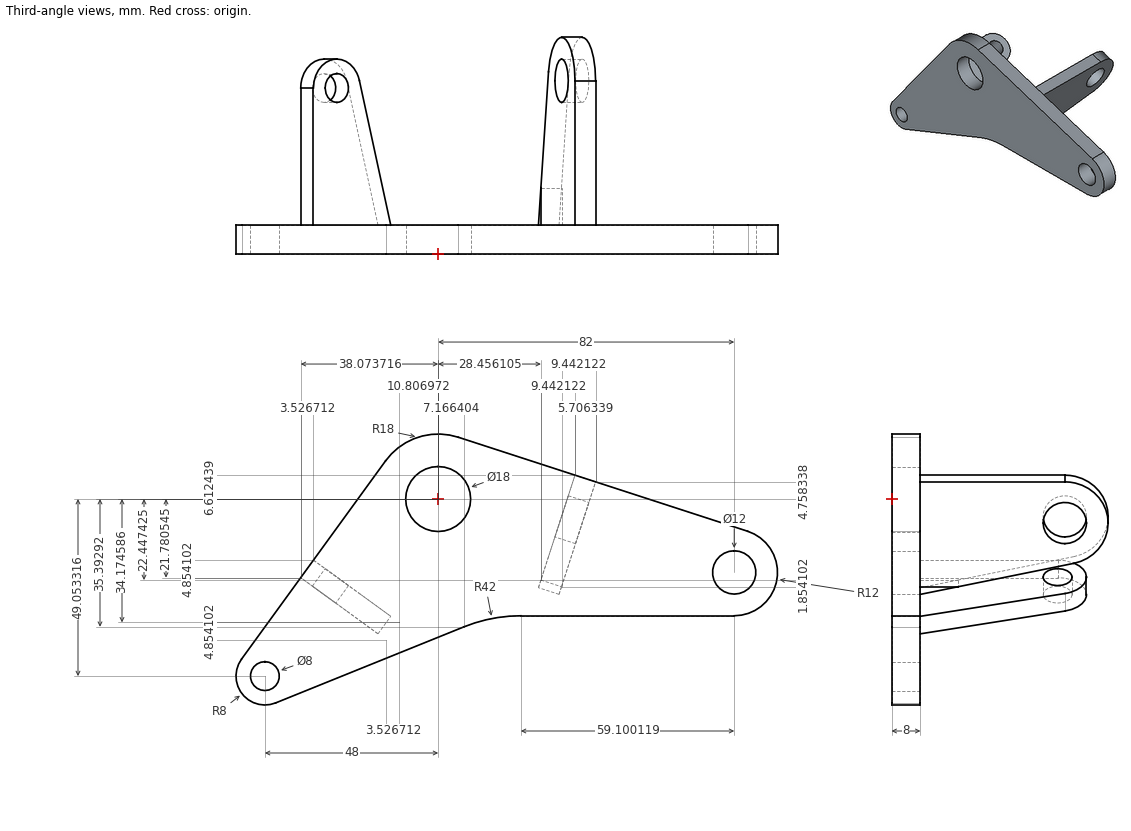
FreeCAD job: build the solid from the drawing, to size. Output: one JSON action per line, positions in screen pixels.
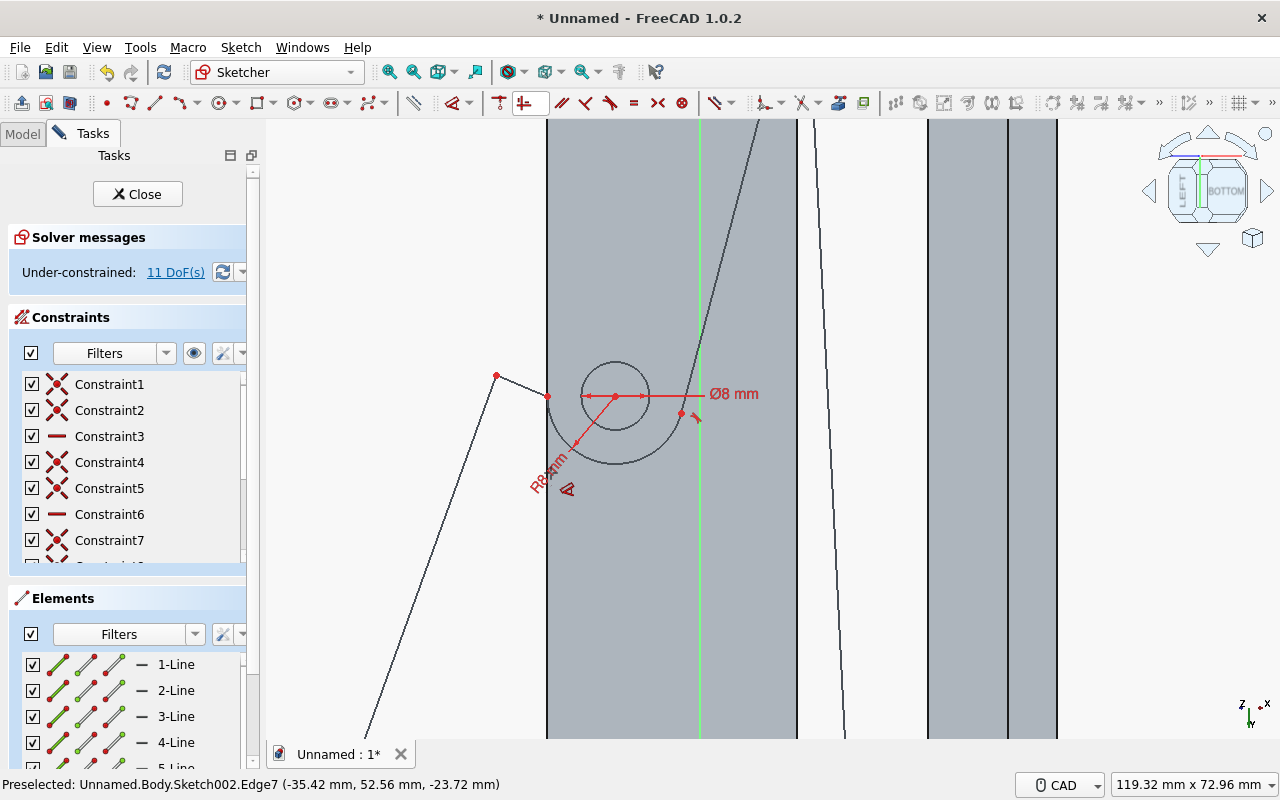
{"action": "scroll", "coordinate": [812, 393], "scroll_direction": "down", "scroll_amount": 4}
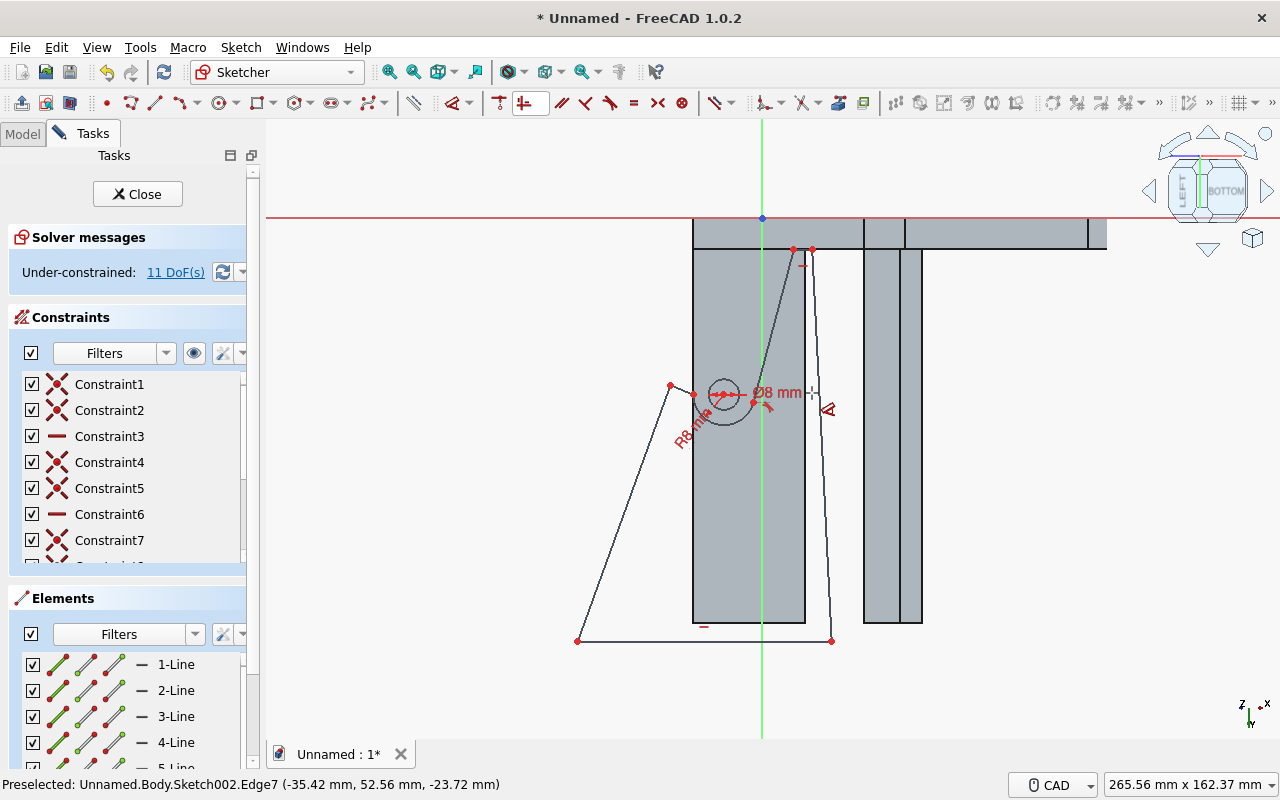
{"action": "scroll", "coordinate": [812, 250], "scroll_direction": "up", "scroll_amount": 2}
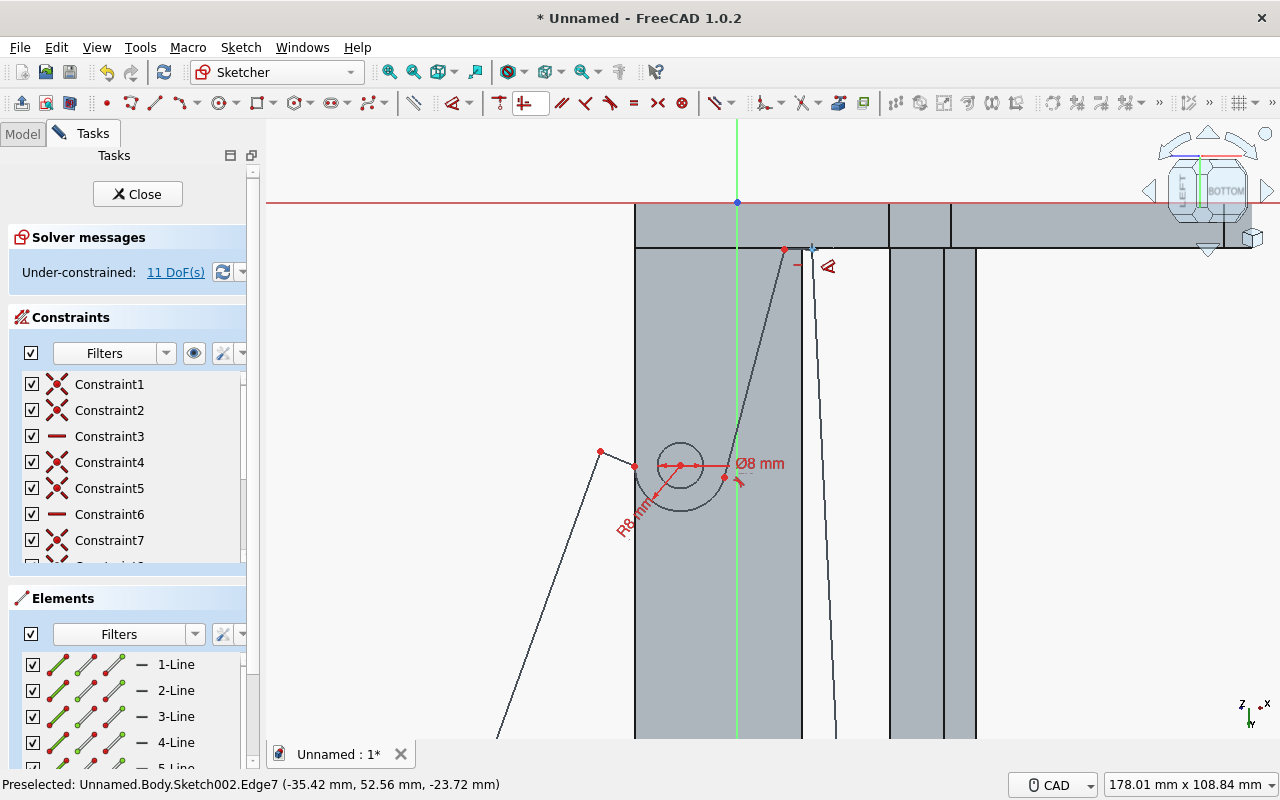
{"action": "left_click", "coordinate": [812, 249]}
{"action": "left_click", "coordinate": [846, 226]}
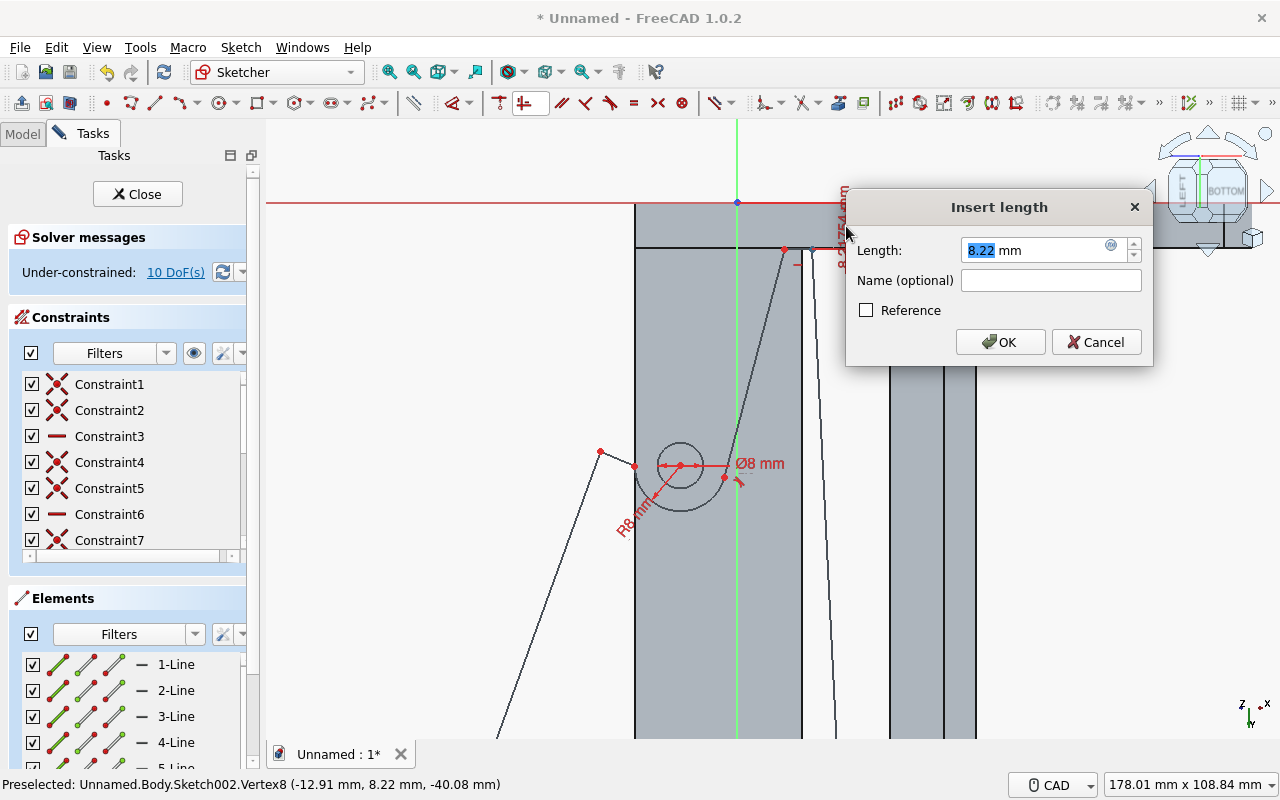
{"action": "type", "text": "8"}
{"action": "key", "text": "Return"}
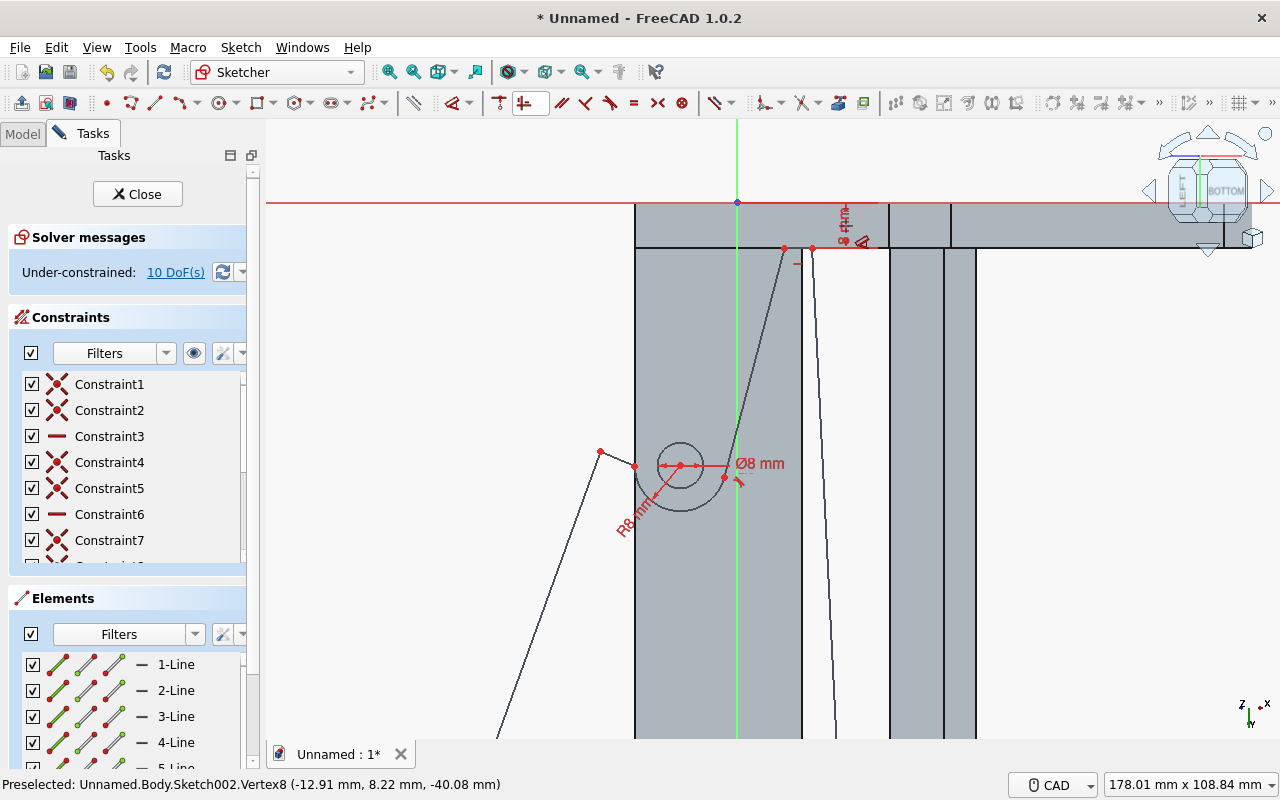
{"action": "left_click", "coordinate": [680, 466]}
{"action": "left_click", "coordinate": [709, 169]}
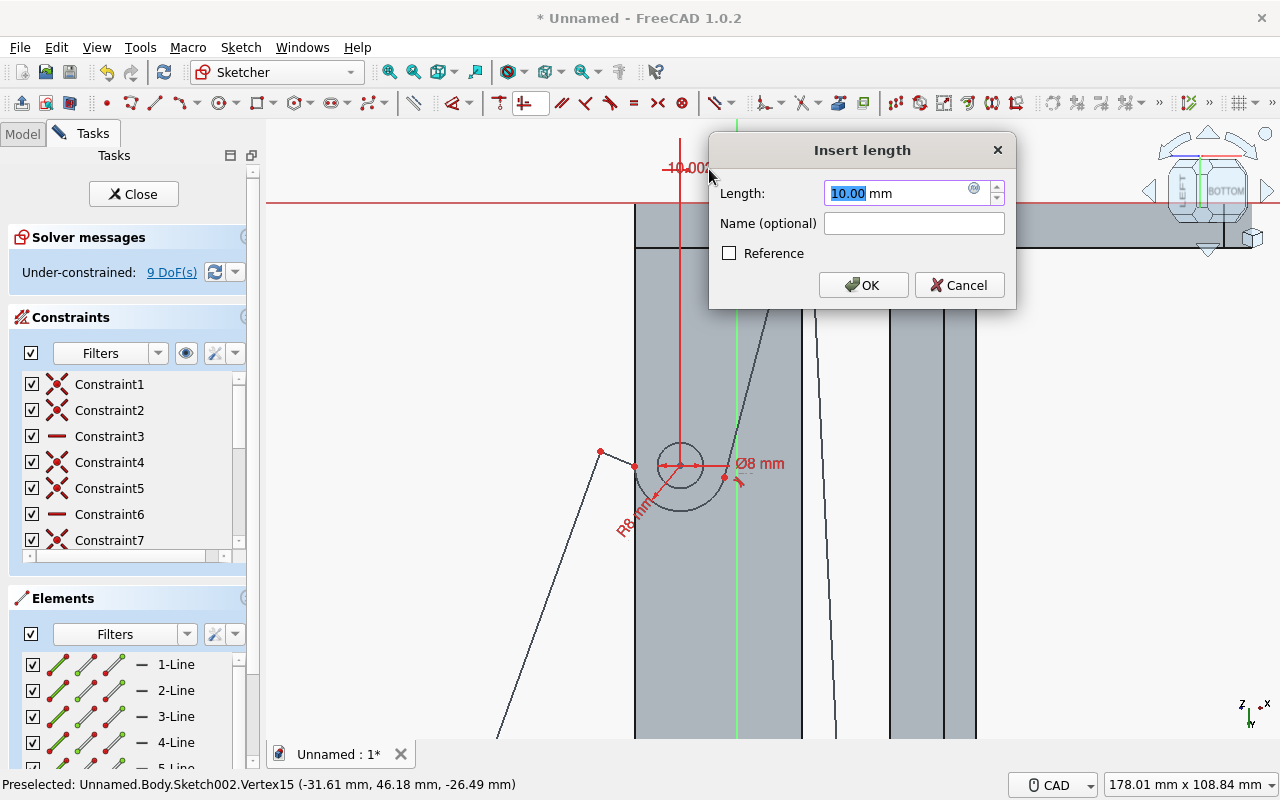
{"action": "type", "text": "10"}
{"action": "key", "text": "Return"}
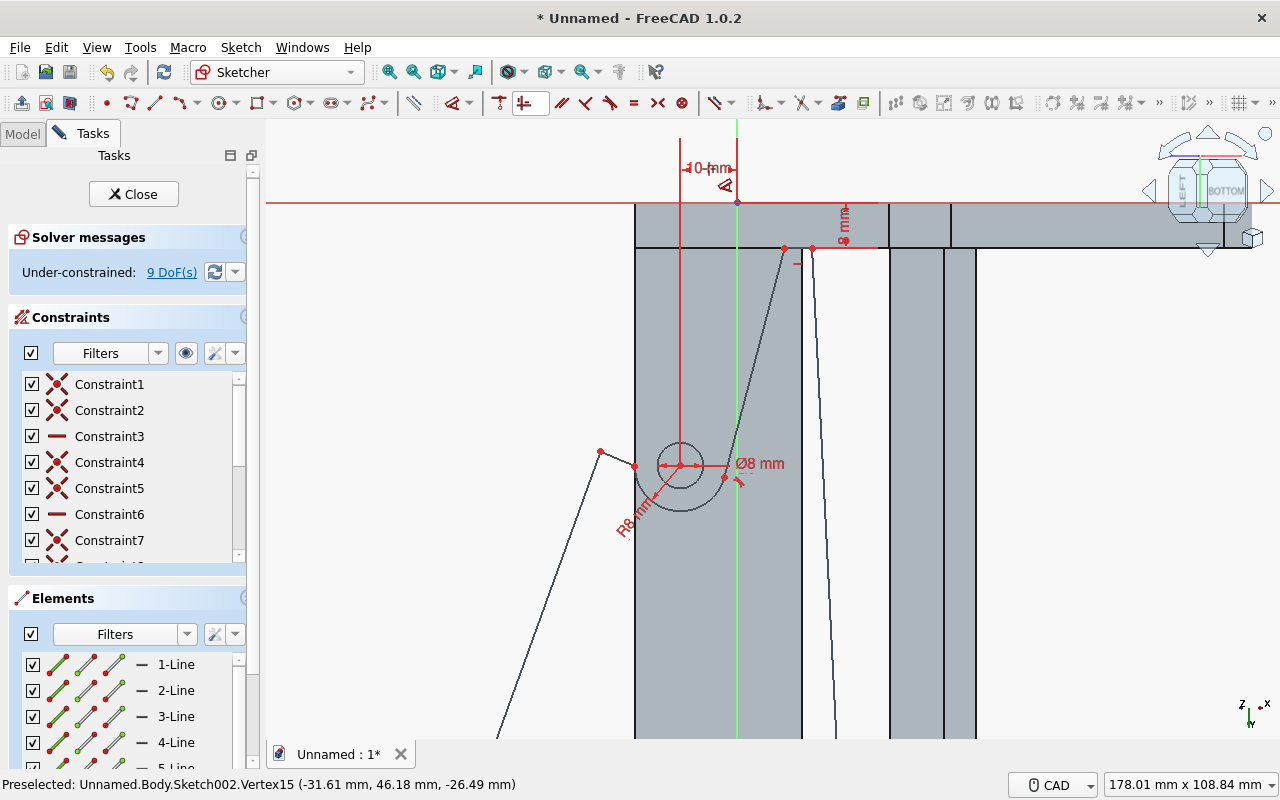
{"action": "left_click", "coordinate": [680, 466]}
{"action": "left_click", "coordinate": [771, 395]}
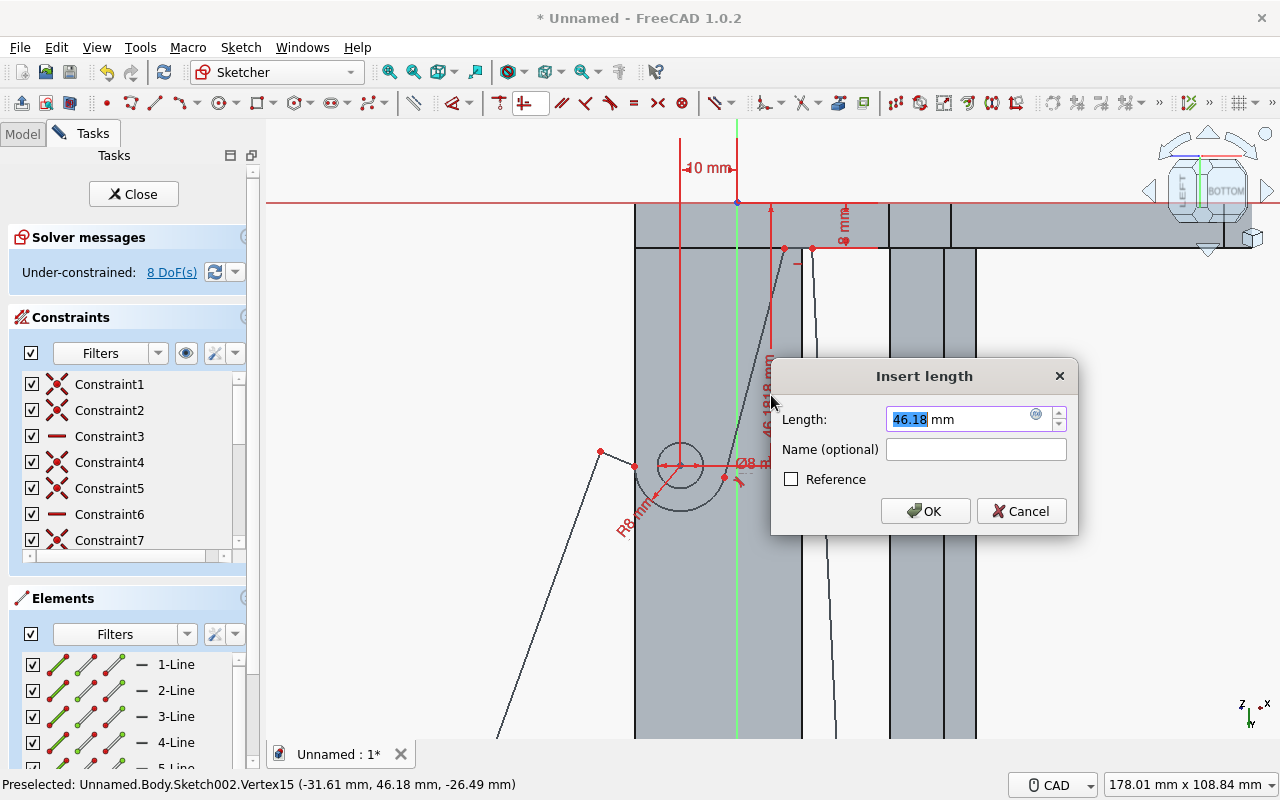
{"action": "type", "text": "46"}
{"action": "key", "text": "Return"}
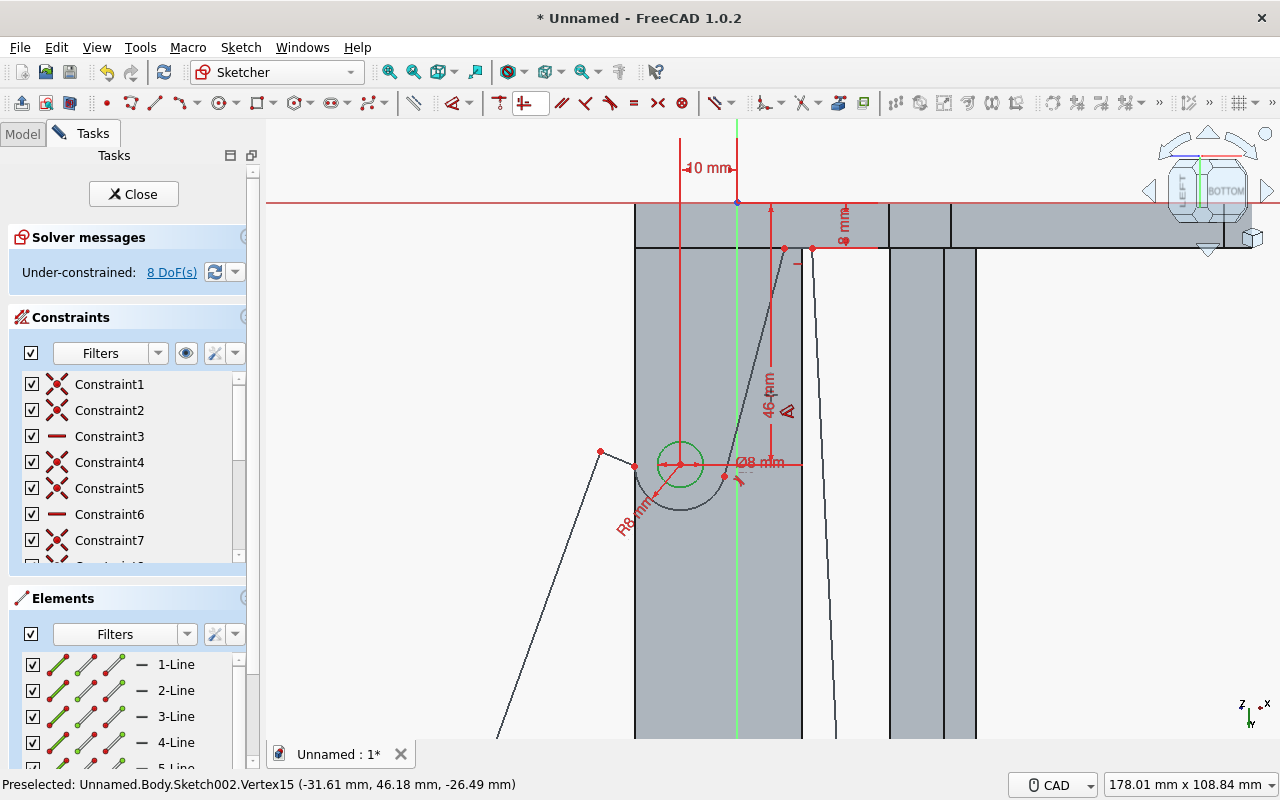
{"action": "left_click", "coordinate": [635, 466]}
{"action": "left_click", "coordinate": [771, 242]}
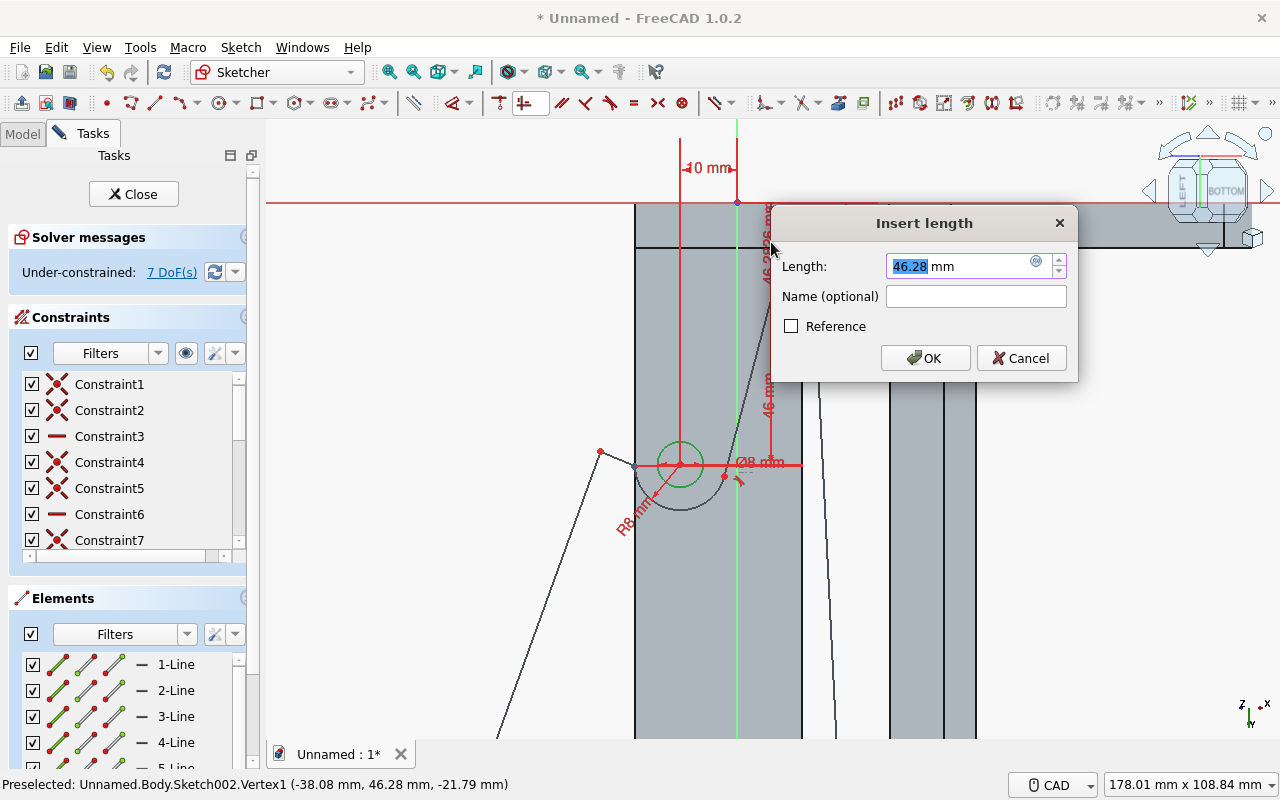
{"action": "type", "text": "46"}
{"action": "key", "text": "Return"}